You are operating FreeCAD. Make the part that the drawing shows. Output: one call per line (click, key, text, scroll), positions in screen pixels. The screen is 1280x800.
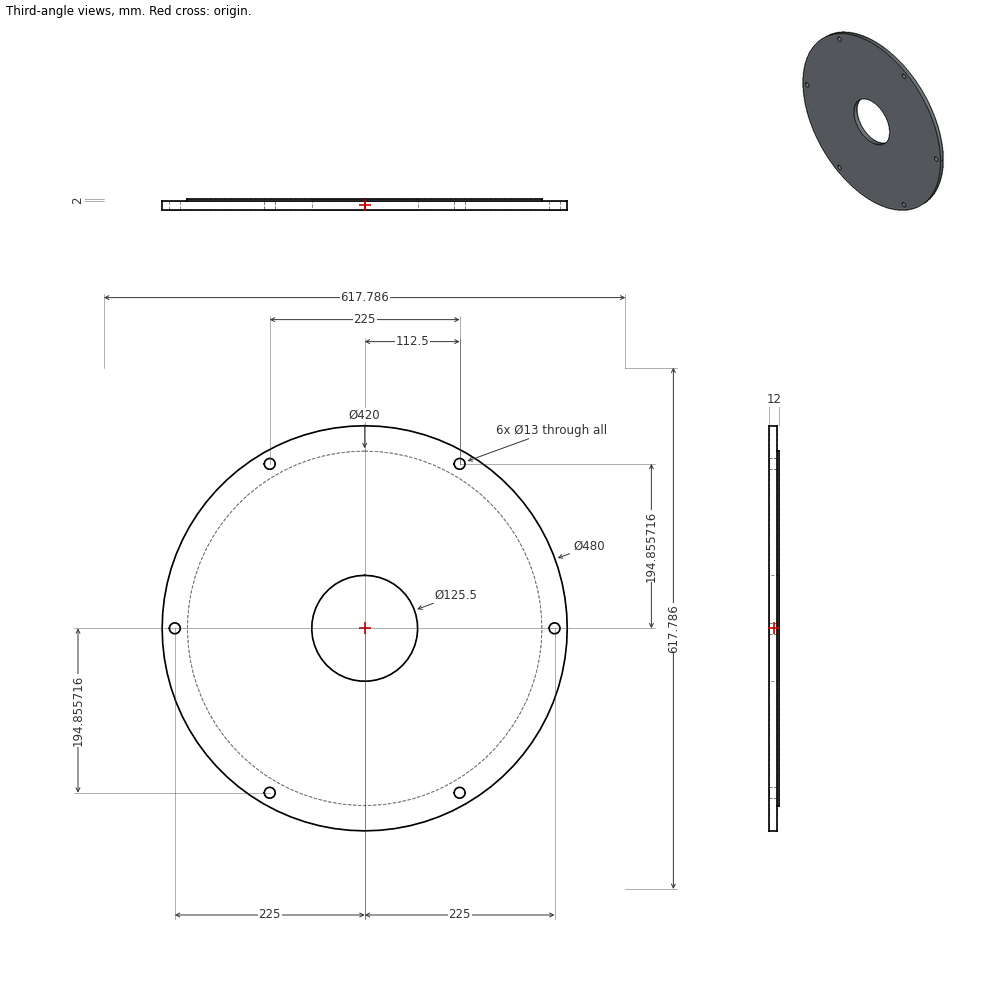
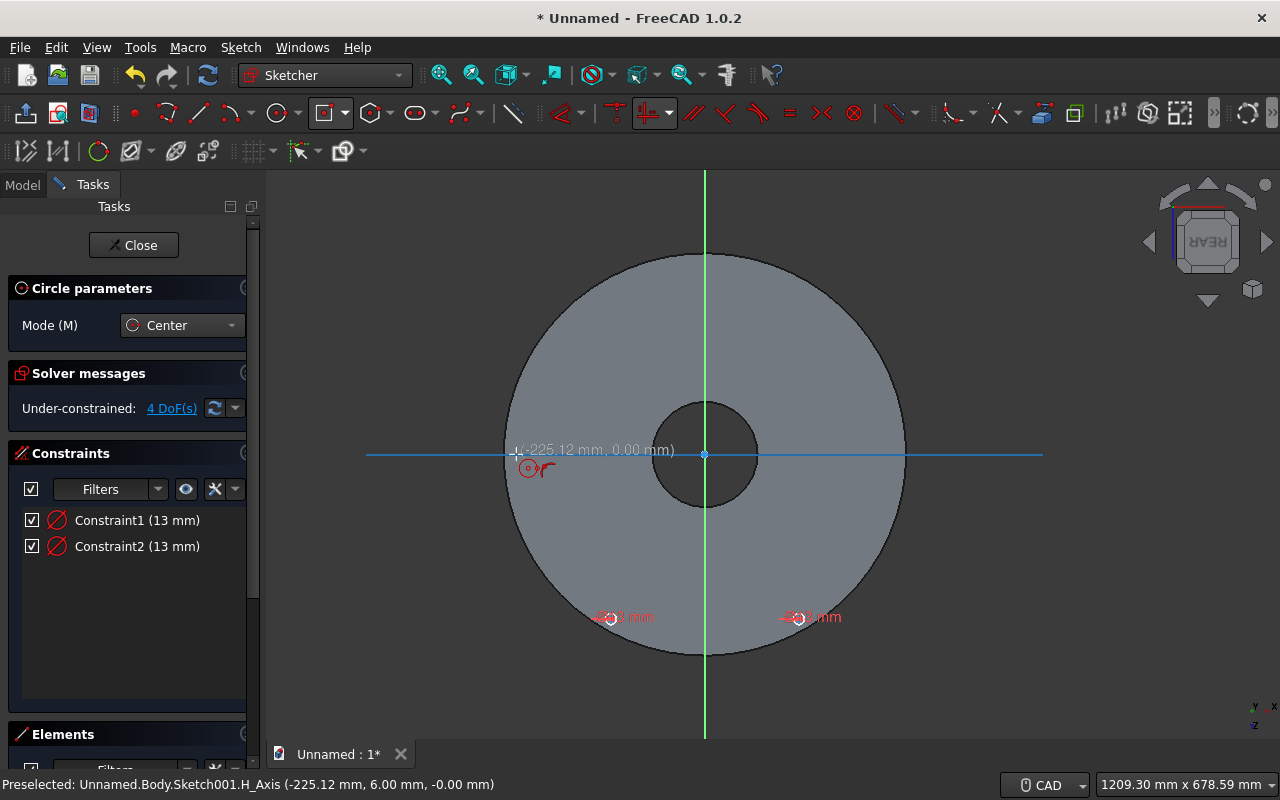
click(516, 455)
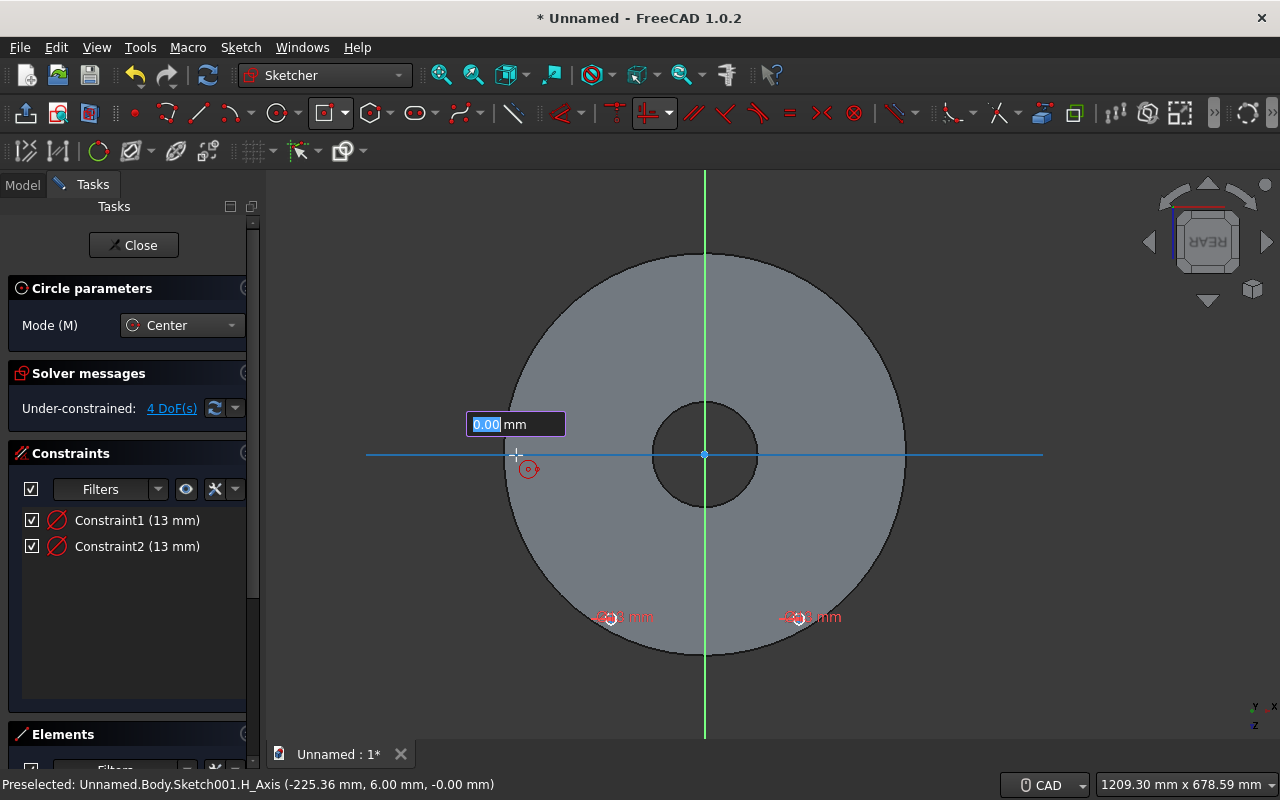
scroll(514, 460, up, 6)
move(515, 458)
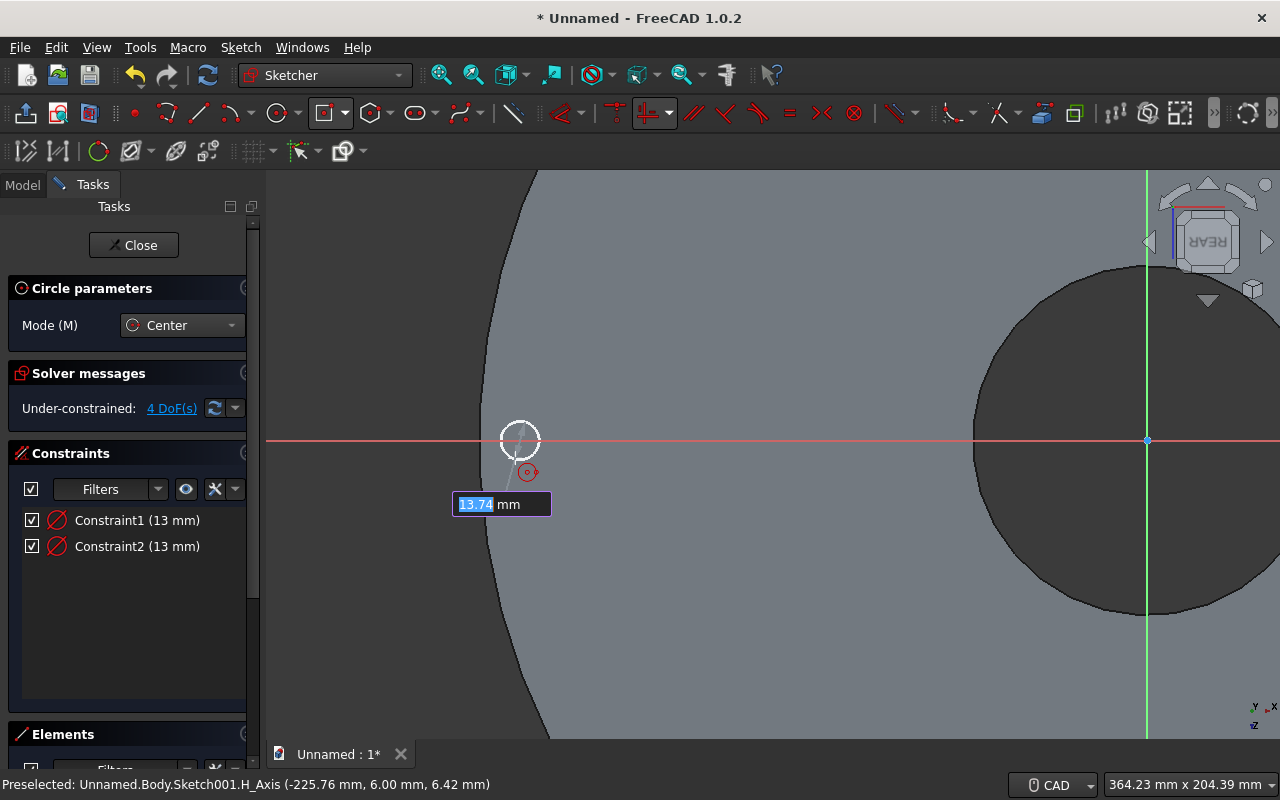
text(13)
key(Return)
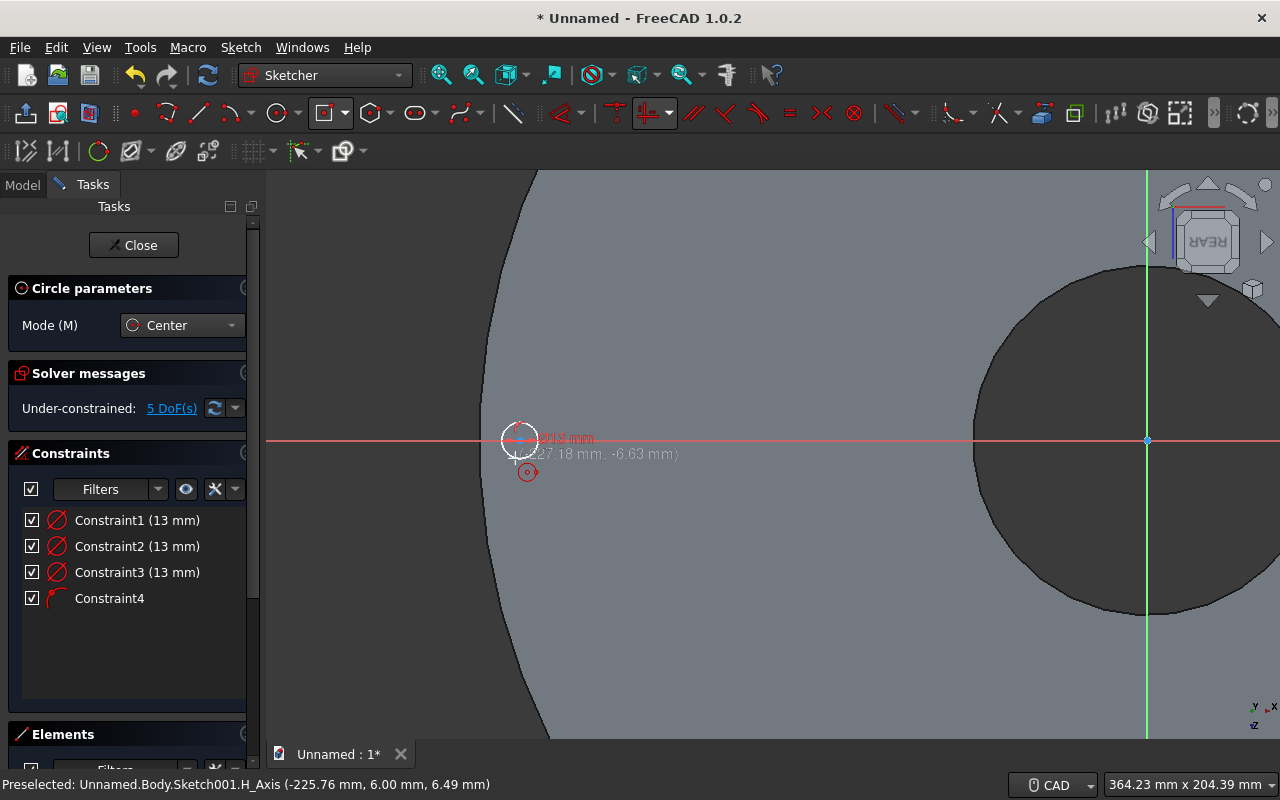
scroll(514, 461, down, 6)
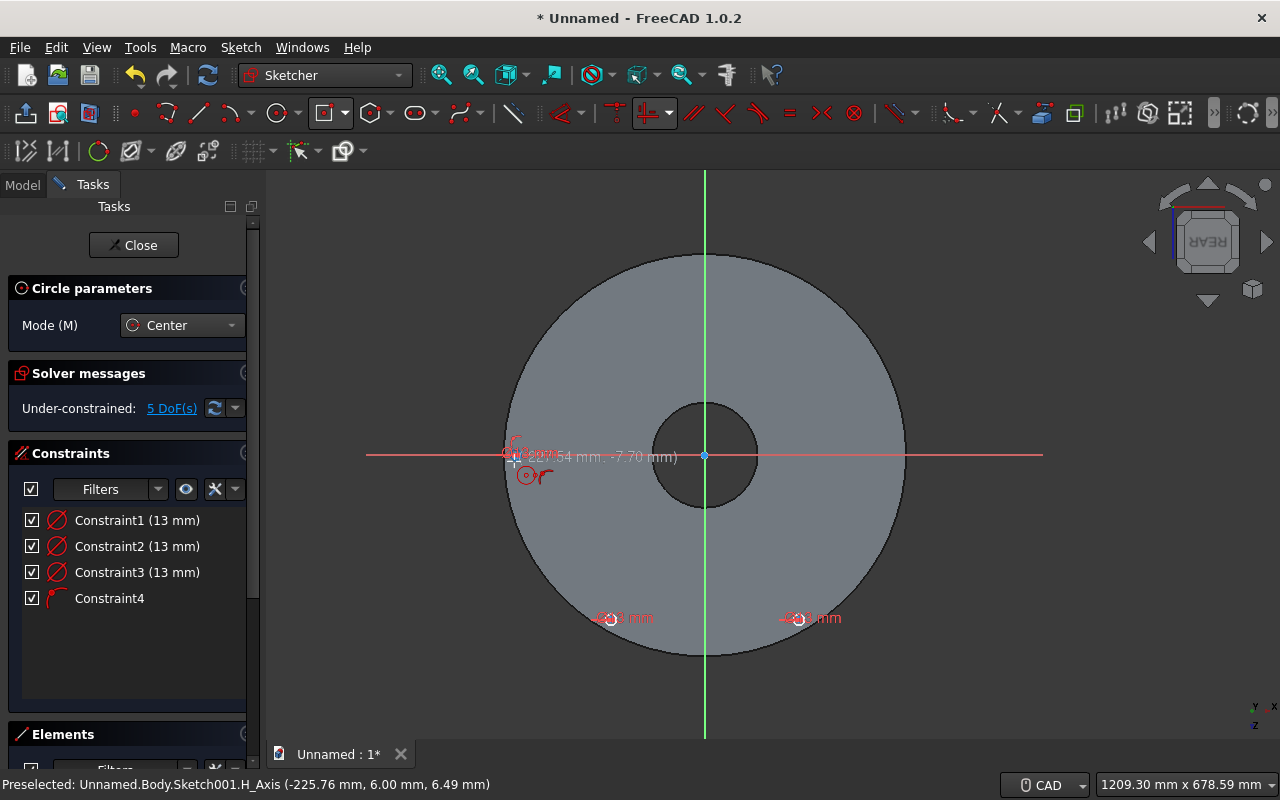
scroll(611, 292, up, 8)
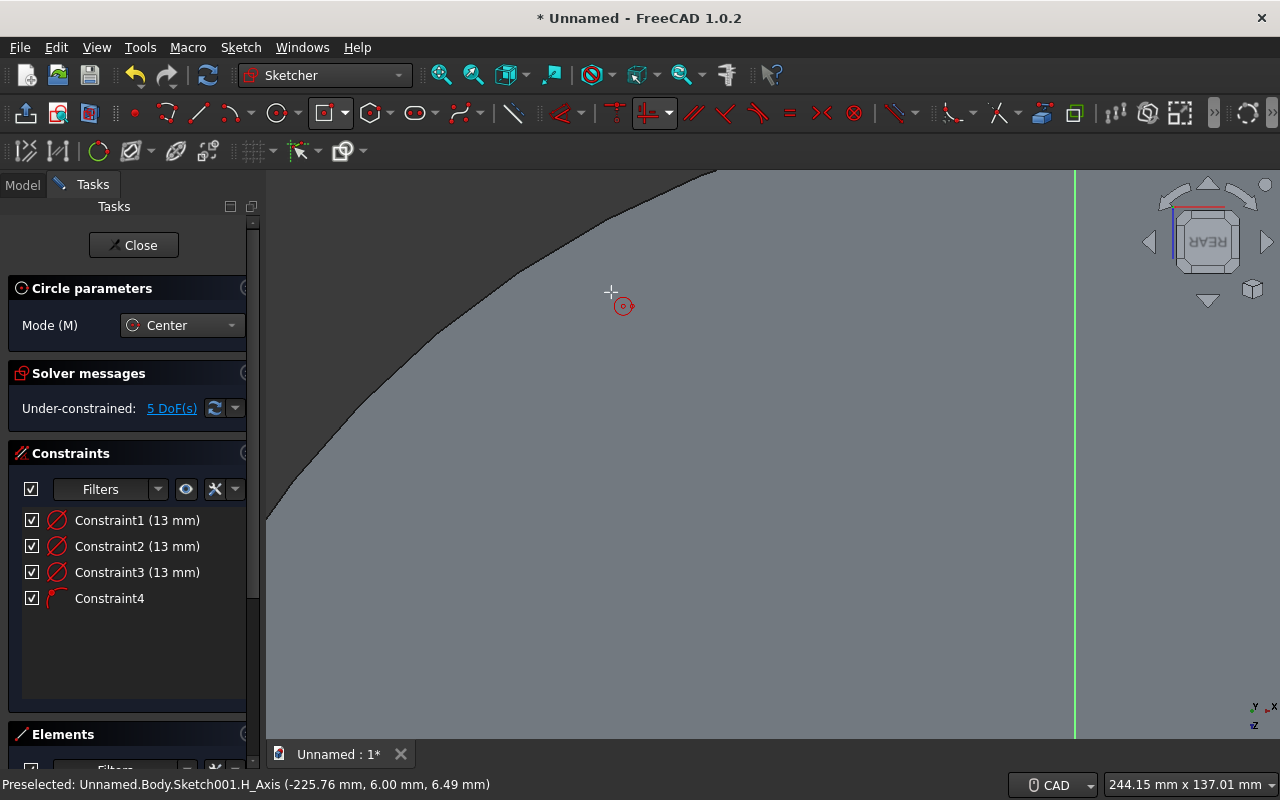
scroll(611, 291, down, 8)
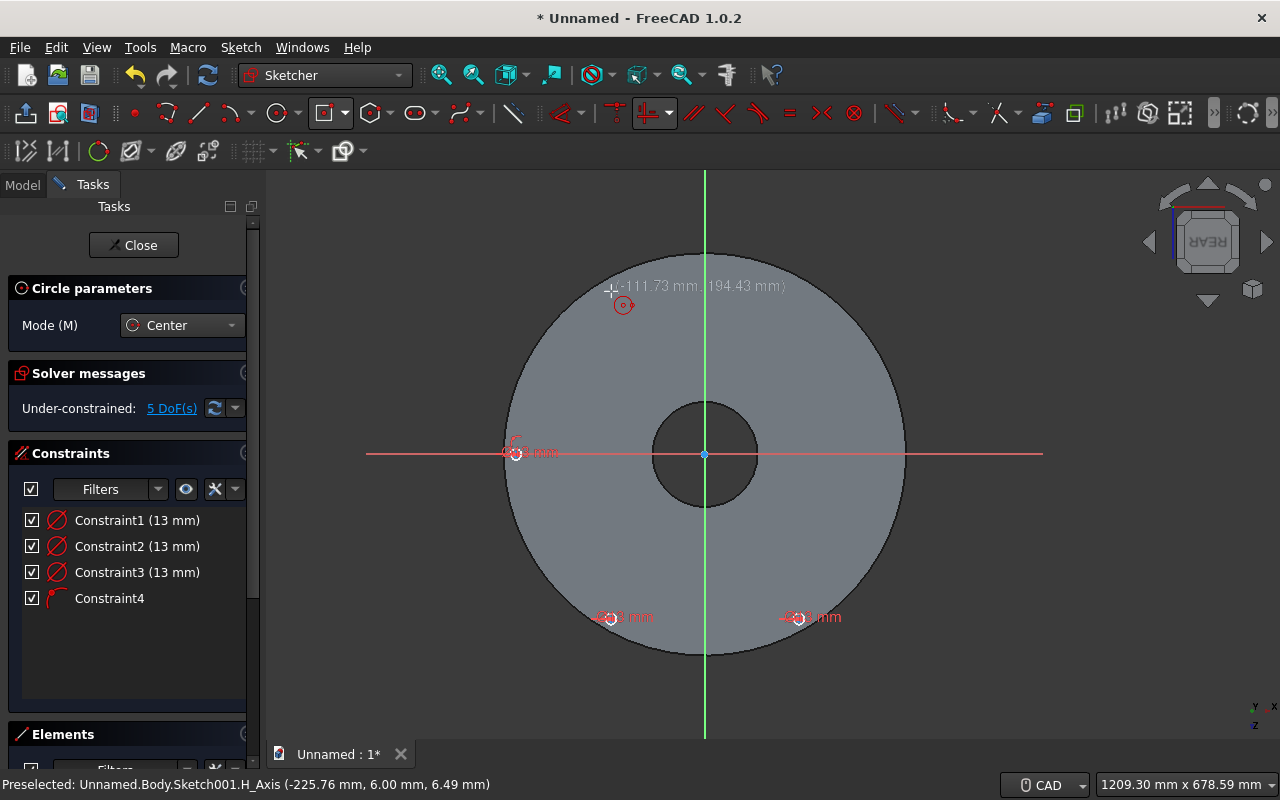
click(611, 291)
move(614, 287)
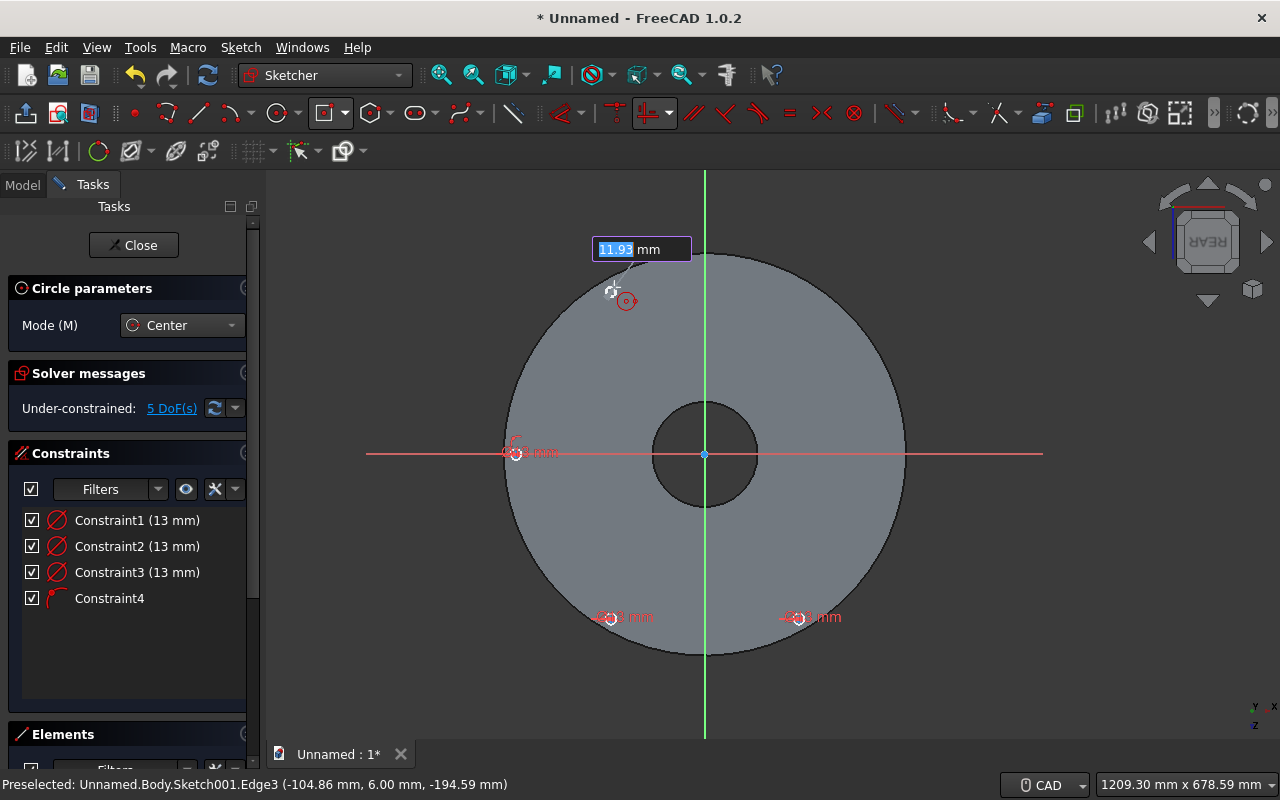
text(13)
key(Return)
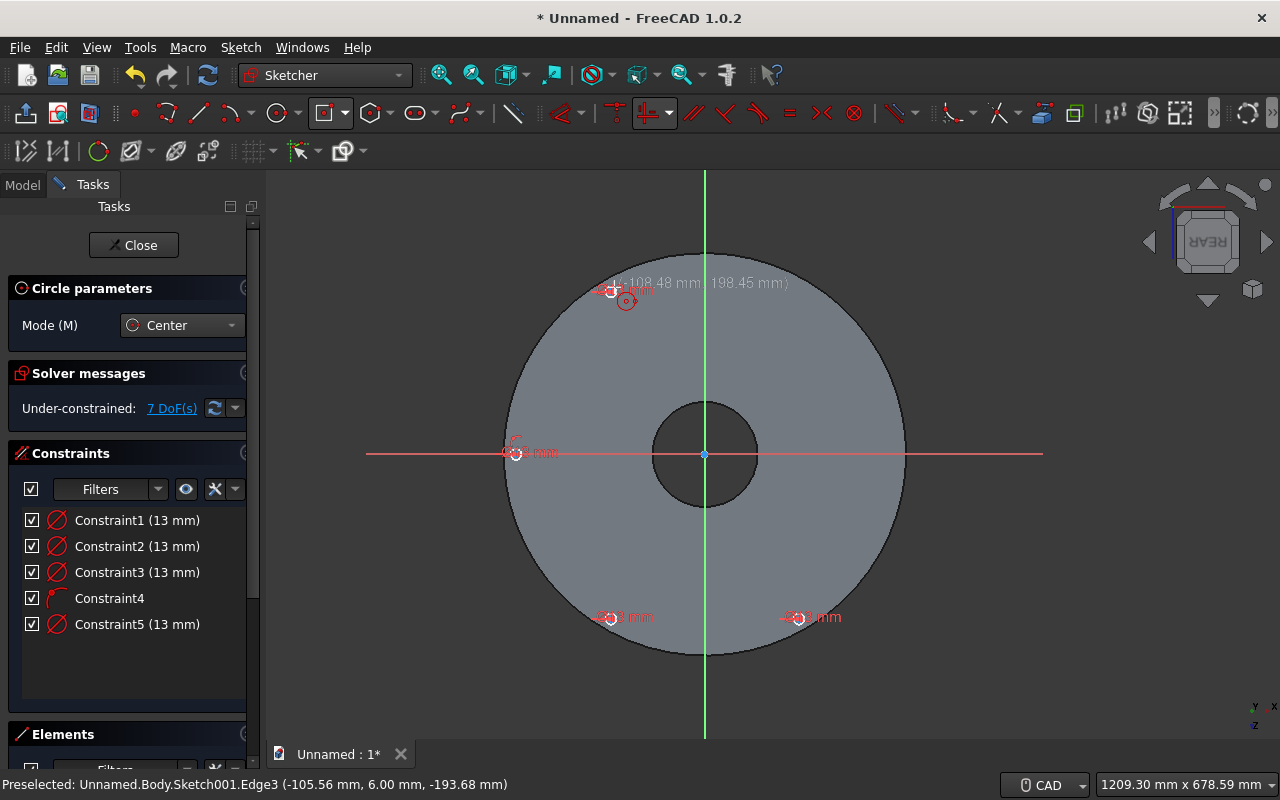
scroll(799, 291, up, 8)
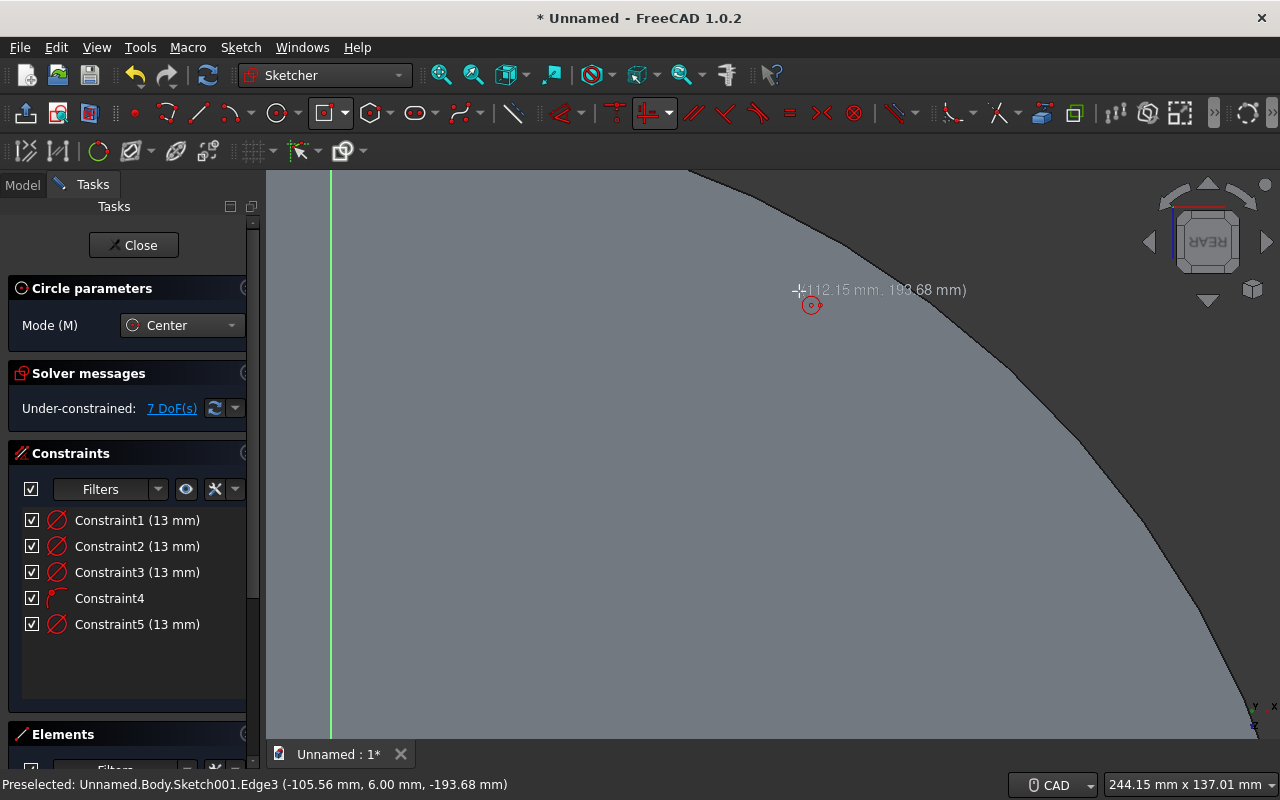
scroll(799, 291, down, 8)